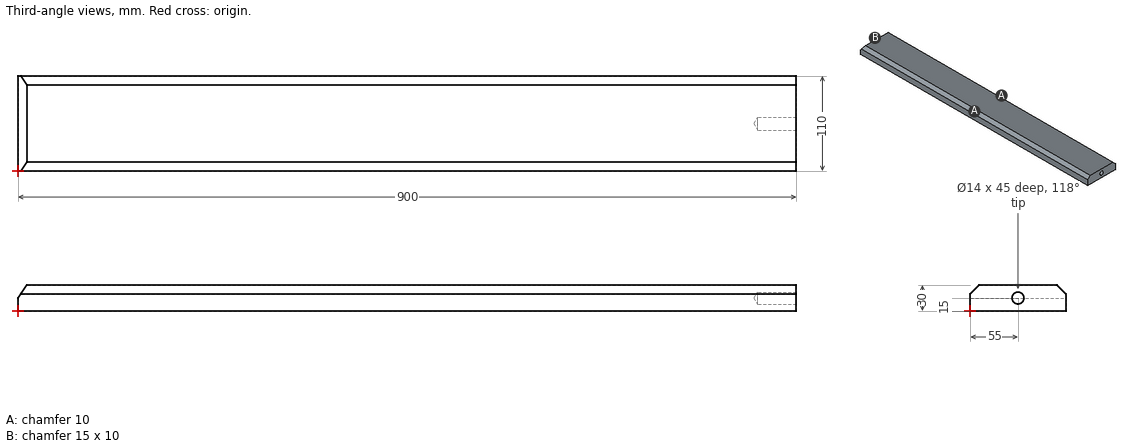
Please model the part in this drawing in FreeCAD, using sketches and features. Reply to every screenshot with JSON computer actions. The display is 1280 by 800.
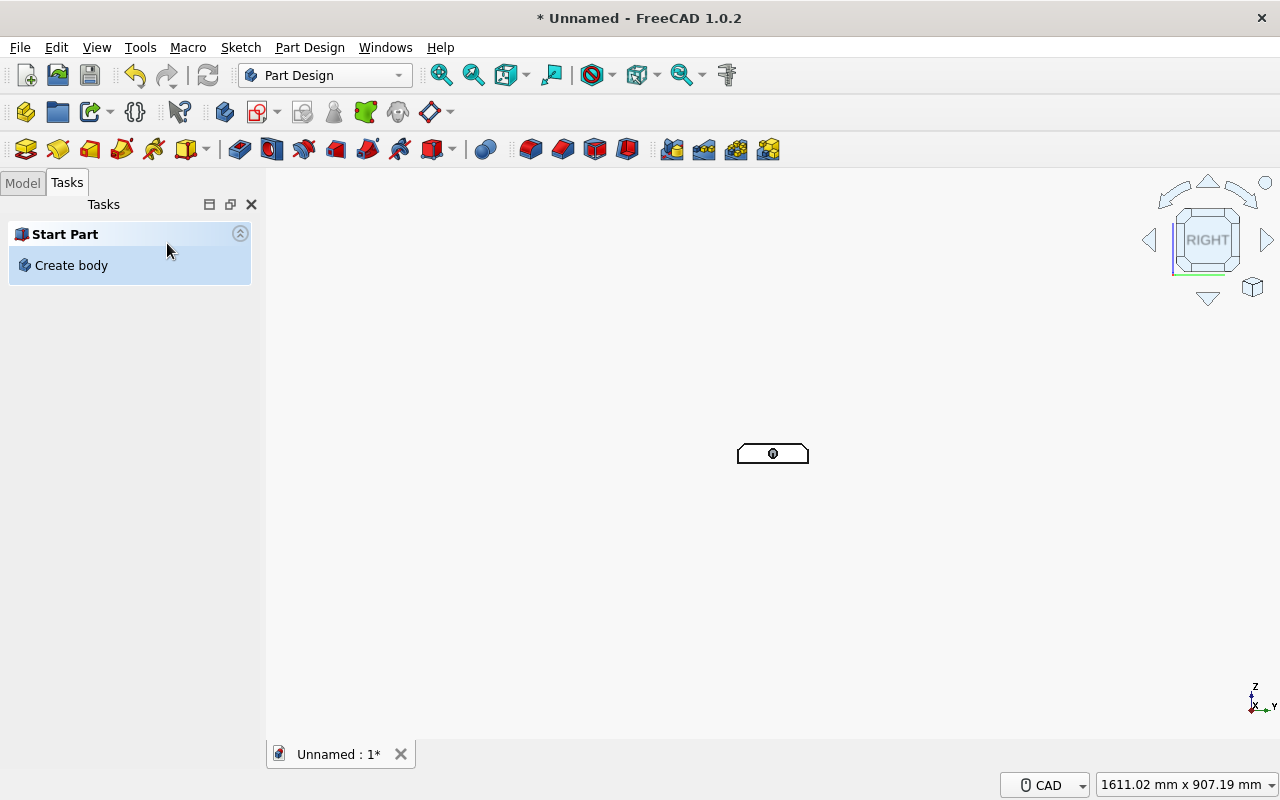
{"action": "key", "text": "0"}